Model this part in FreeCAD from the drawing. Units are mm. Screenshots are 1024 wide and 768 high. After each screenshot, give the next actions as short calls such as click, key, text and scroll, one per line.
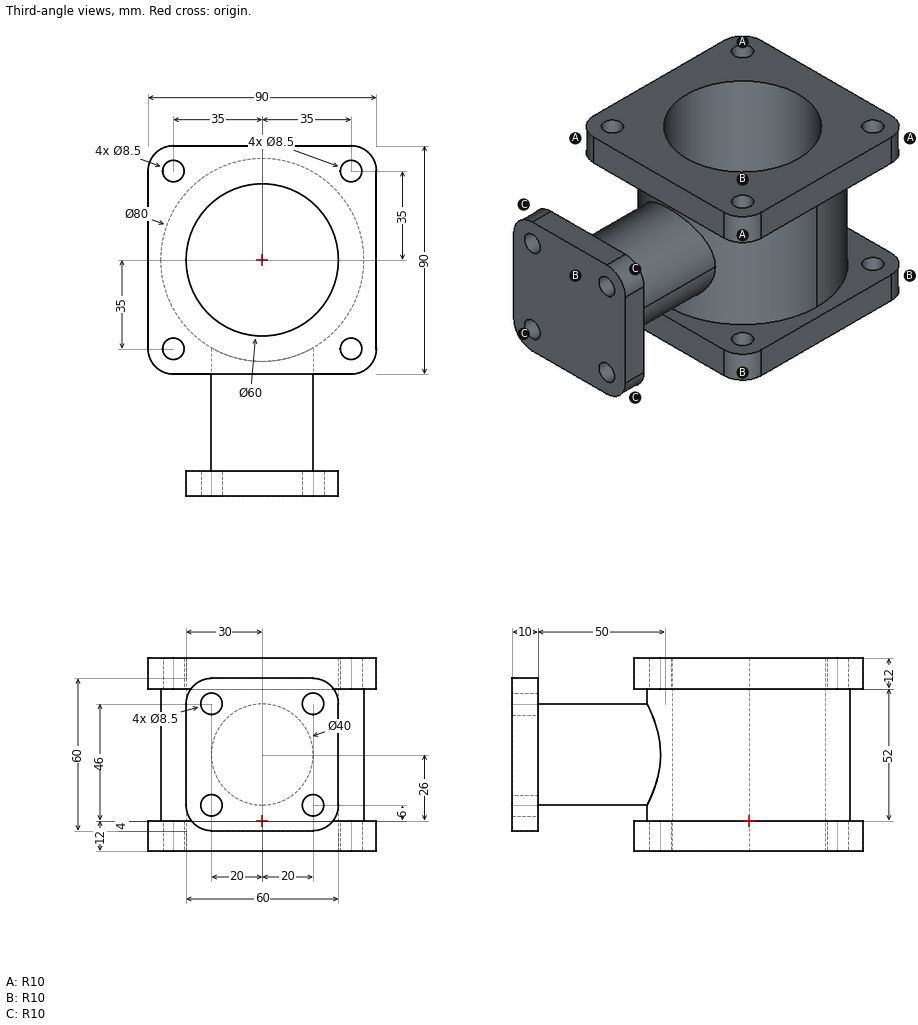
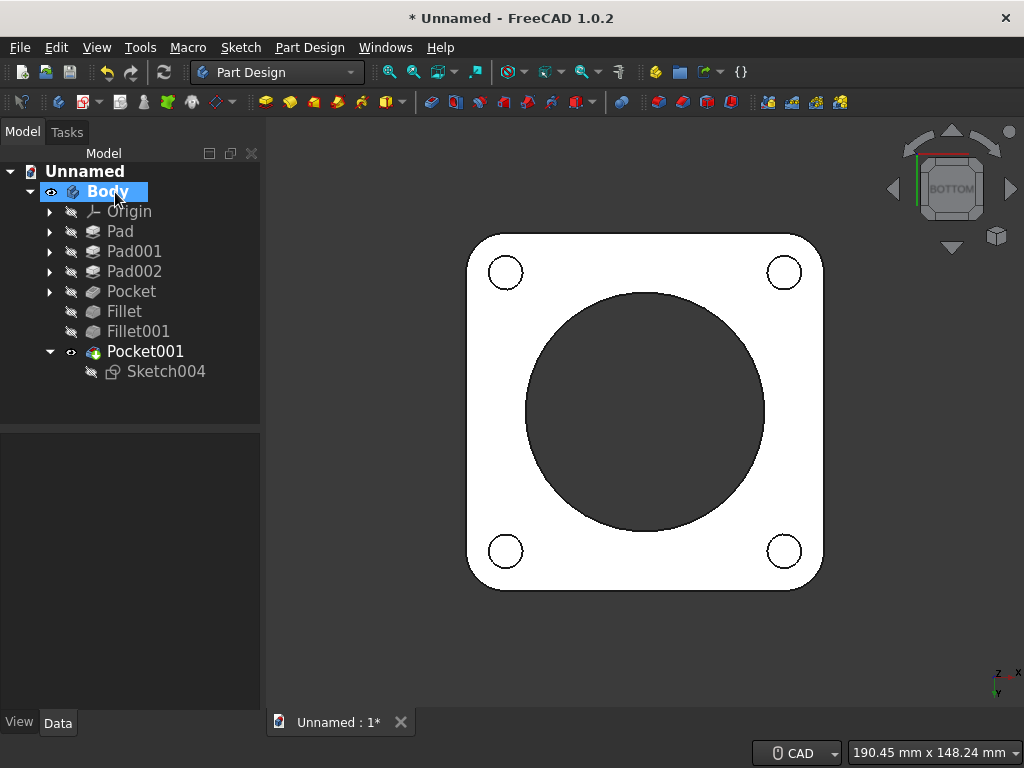
click(50, 212)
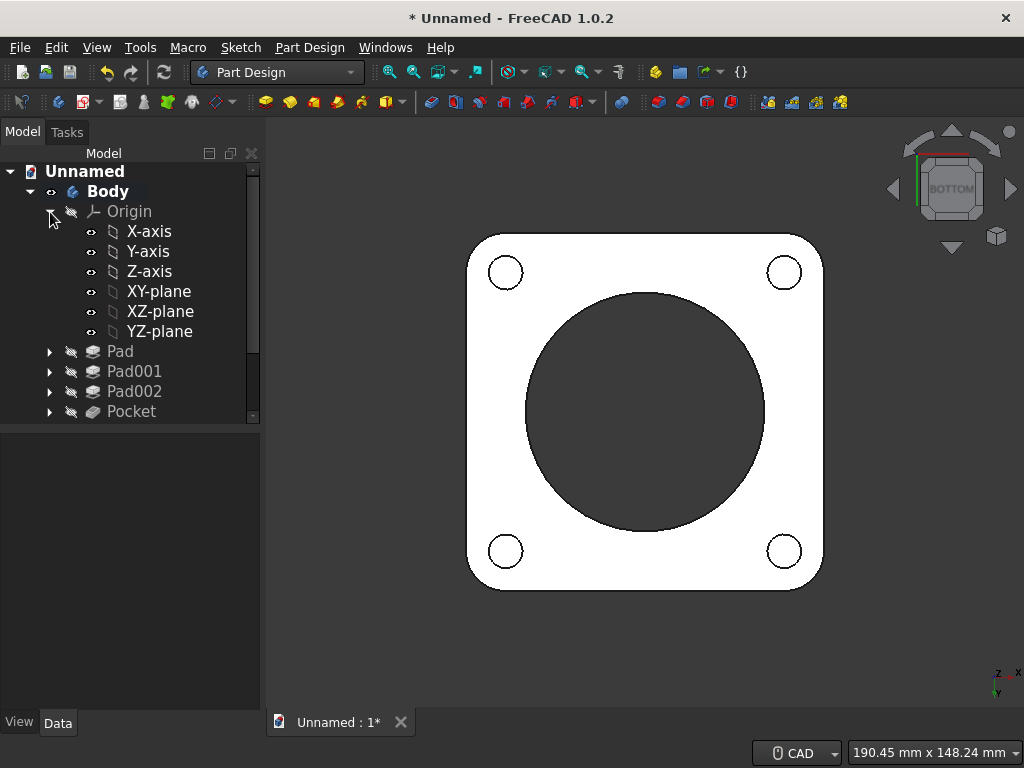
click(136, 292)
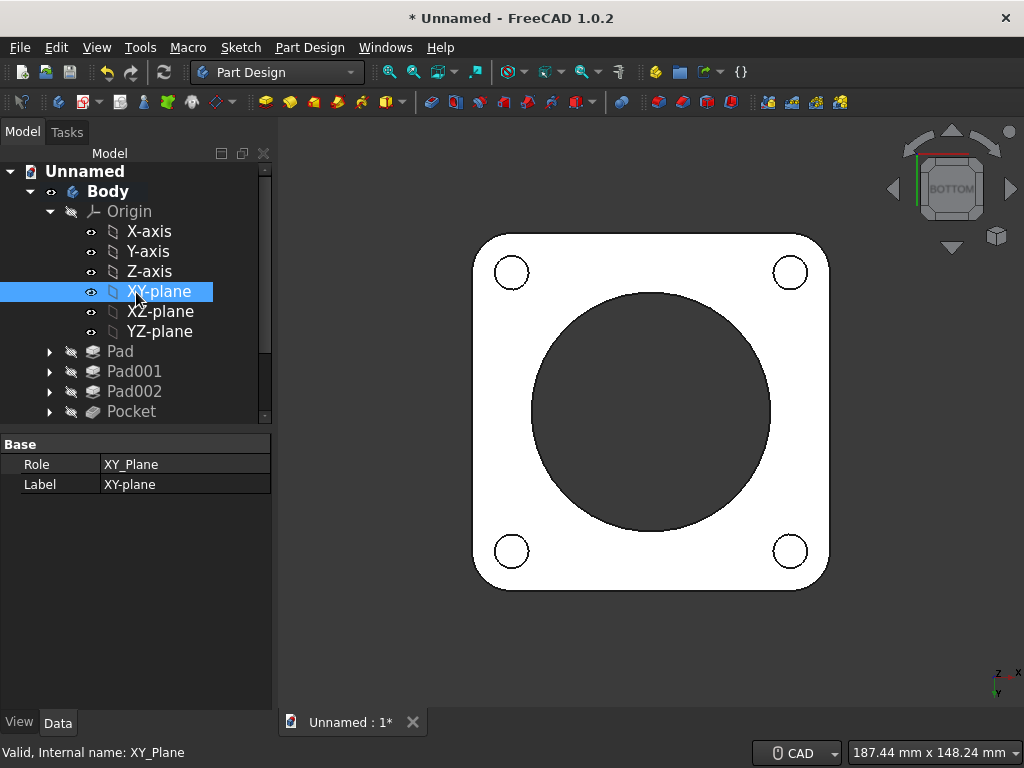
click(216, 102)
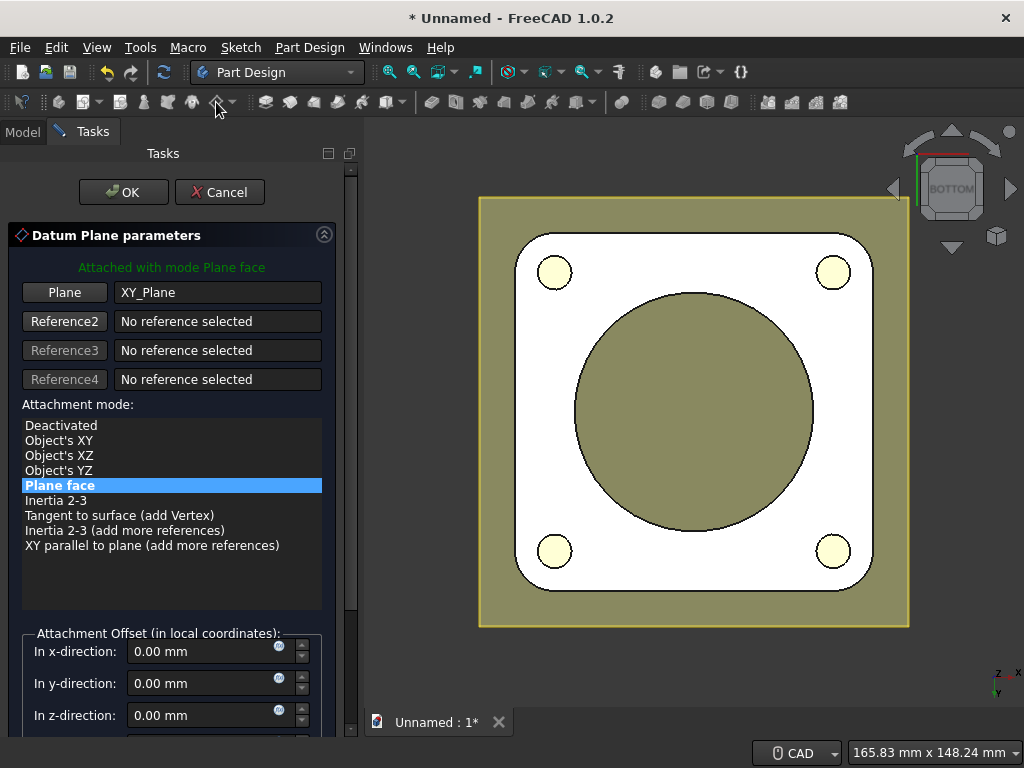
triple_click(210, 715)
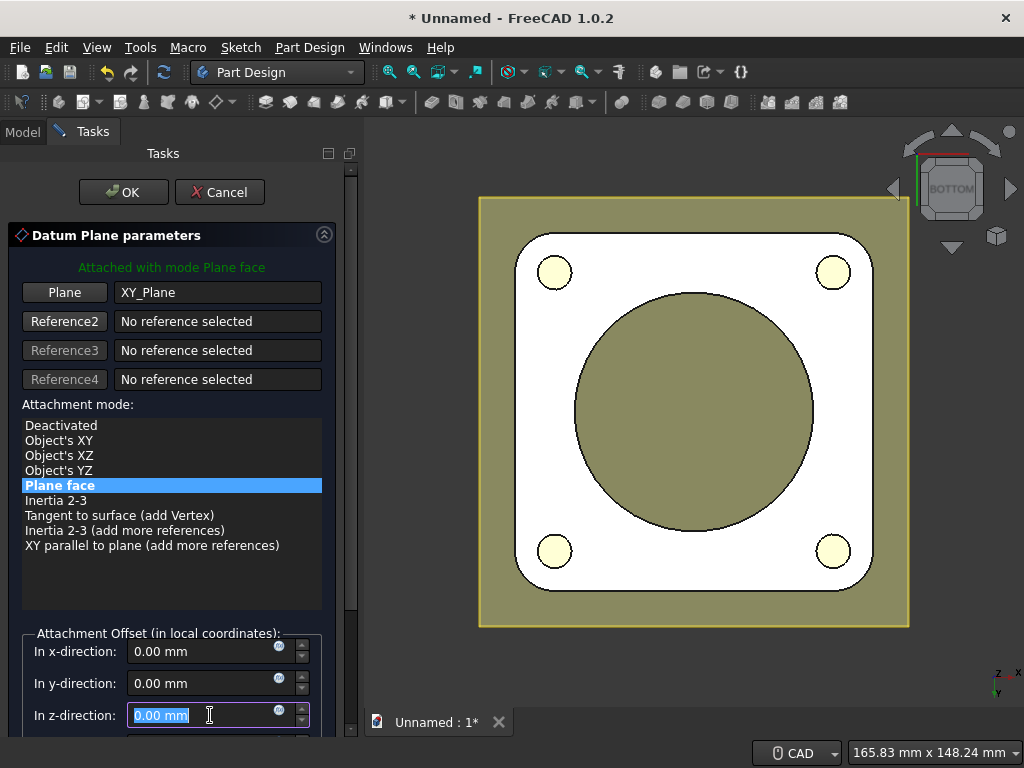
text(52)
key(Tab)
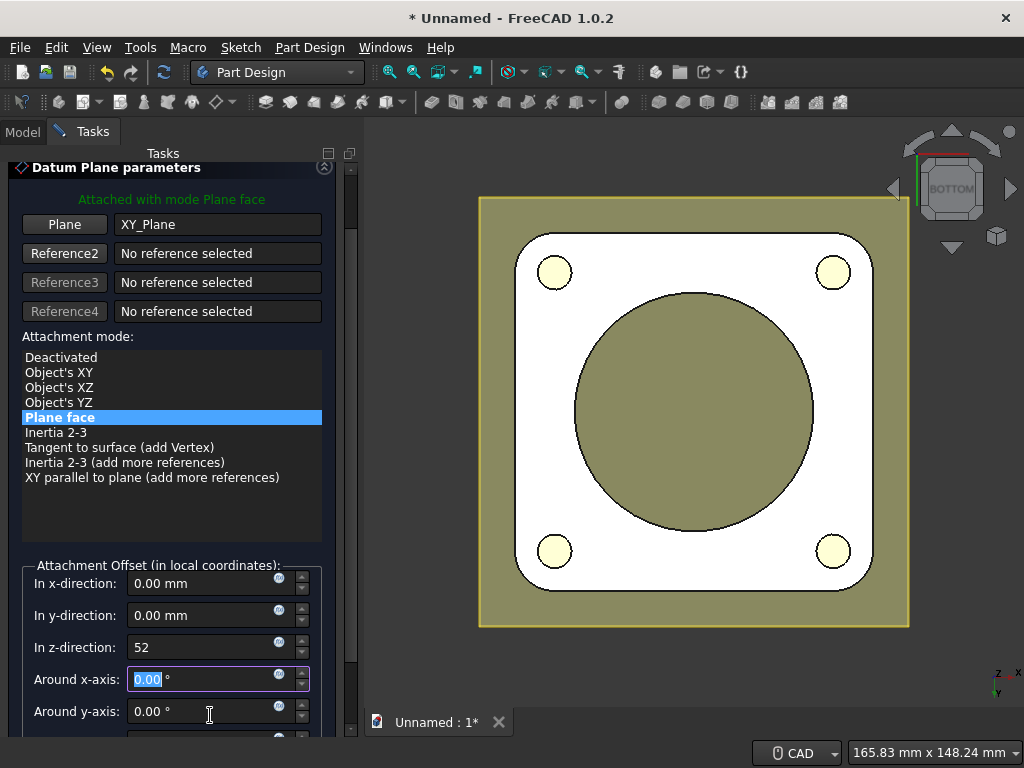
scroll(351, 450, up, 2)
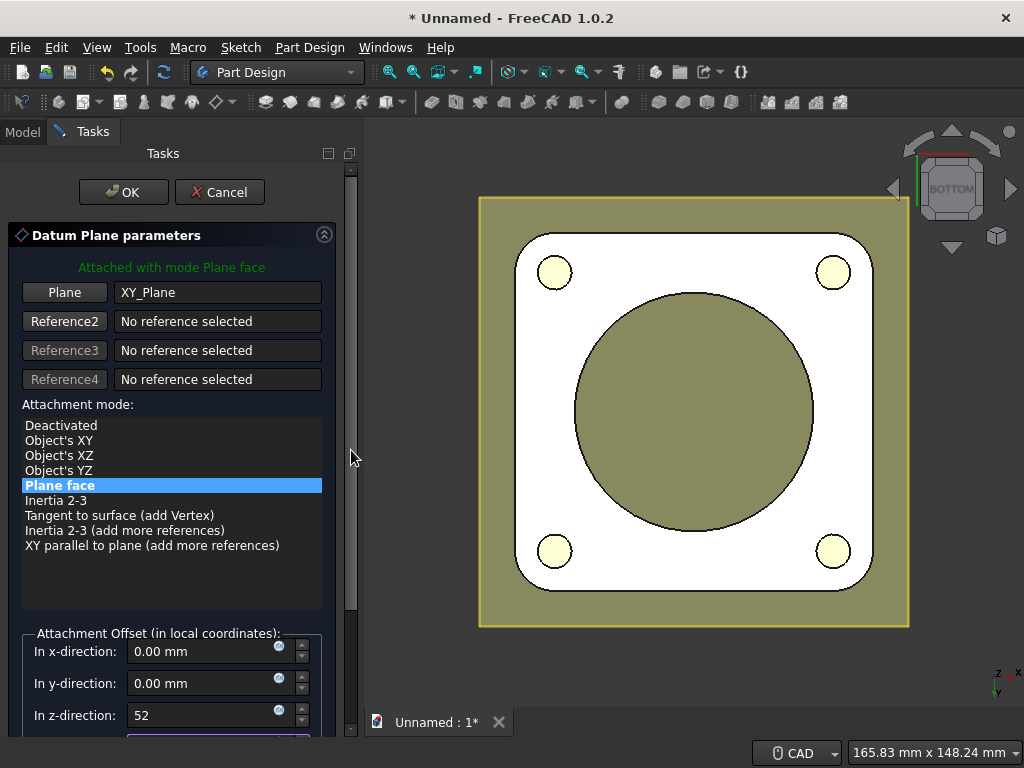
click(124, 192)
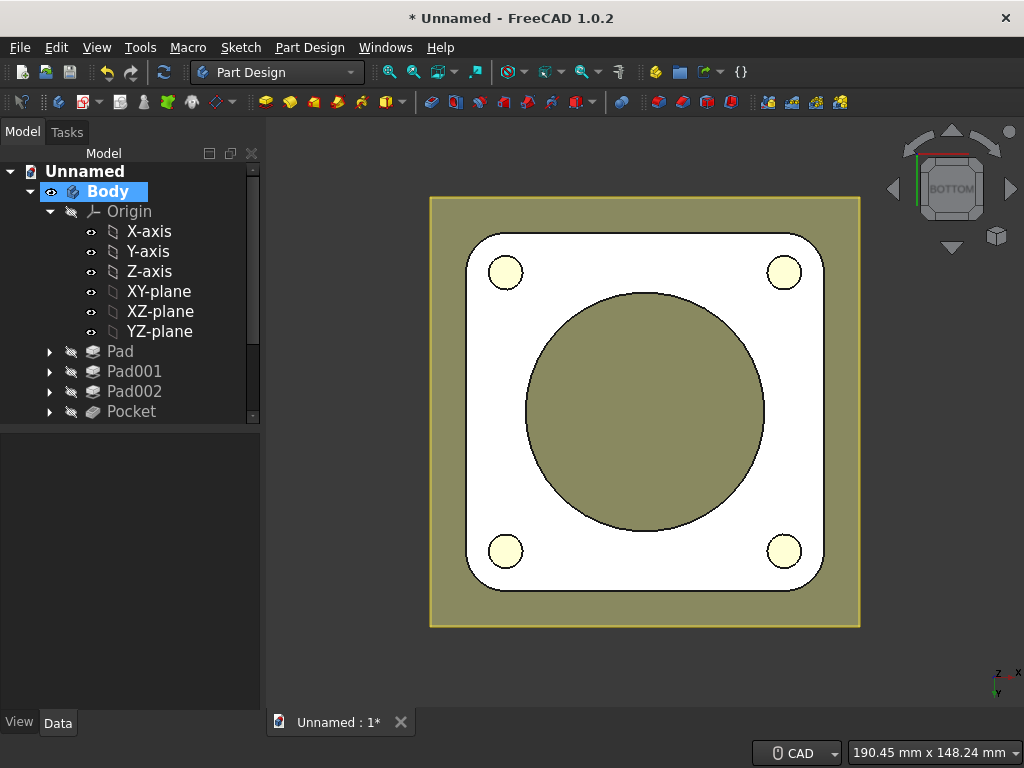
scroll(100, 287, down, 3)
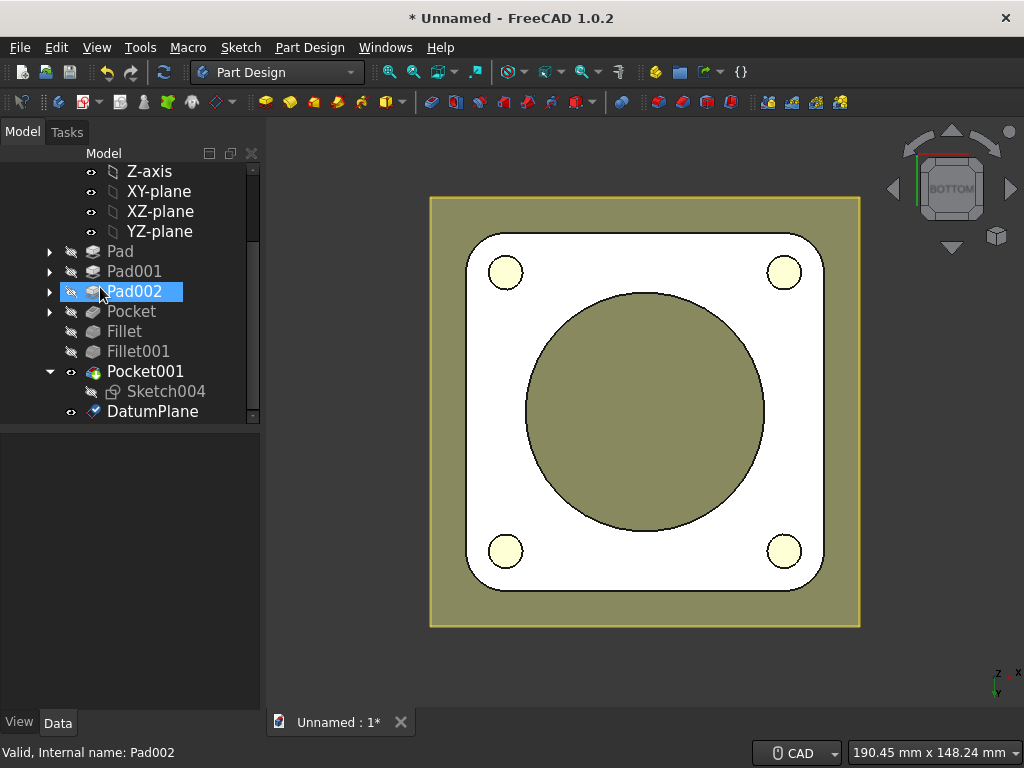
click(116, 412)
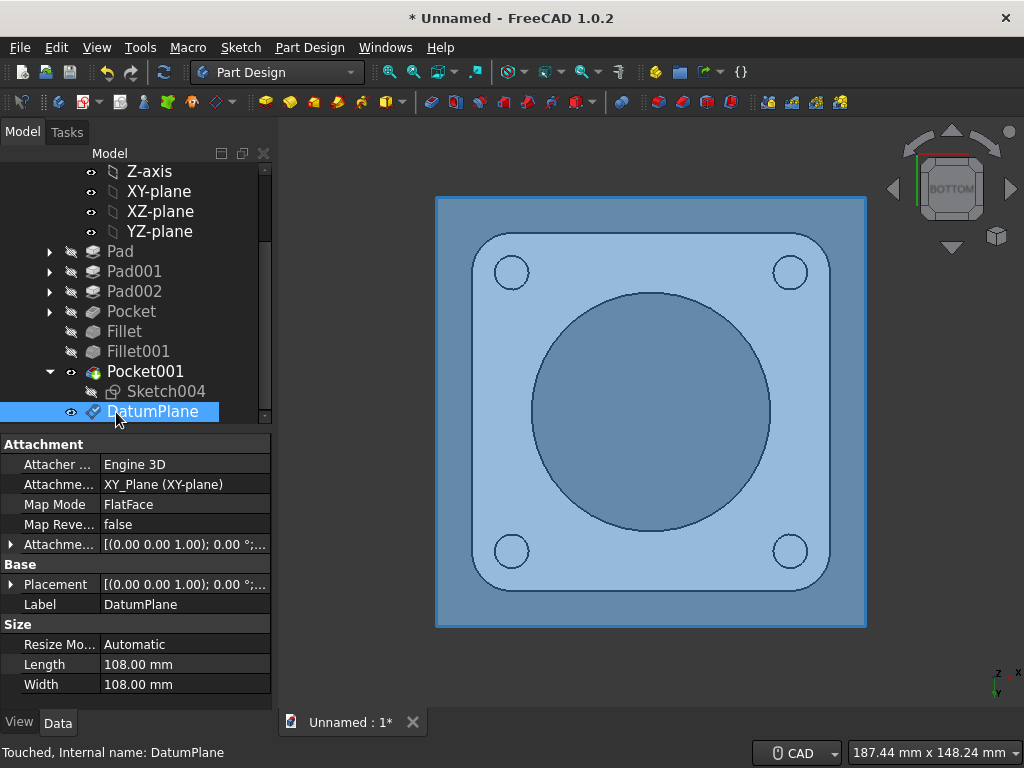
click(84, 102)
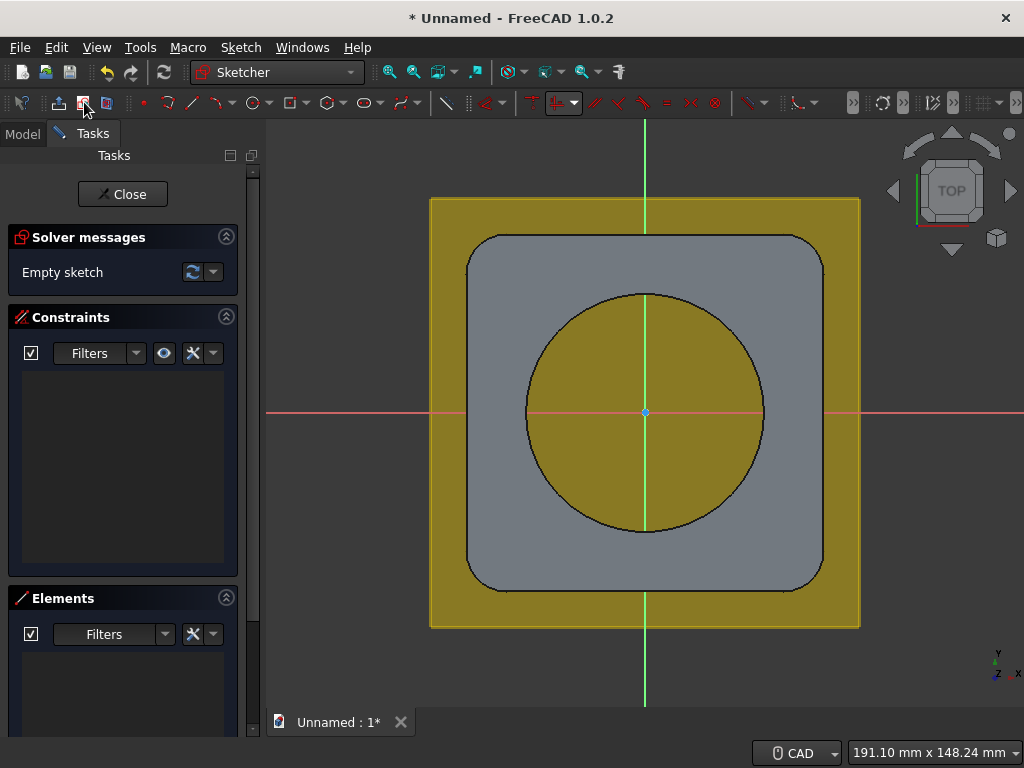
click(108, 104)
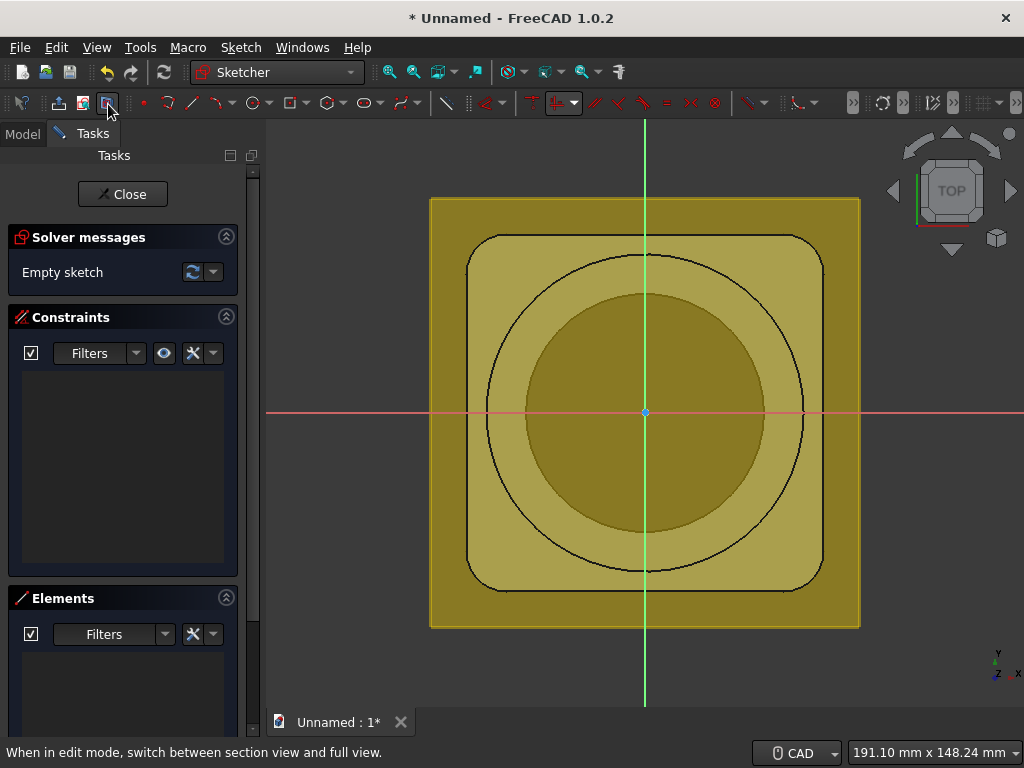
click(254, 104)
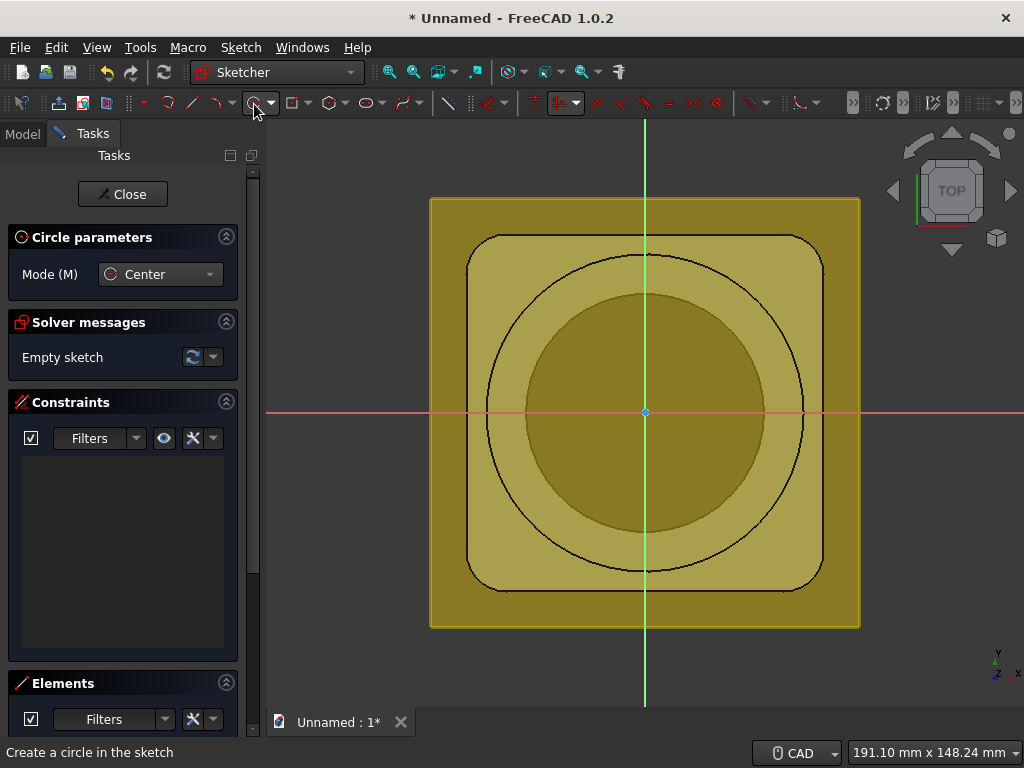
scroll(506, 274, up, 2)